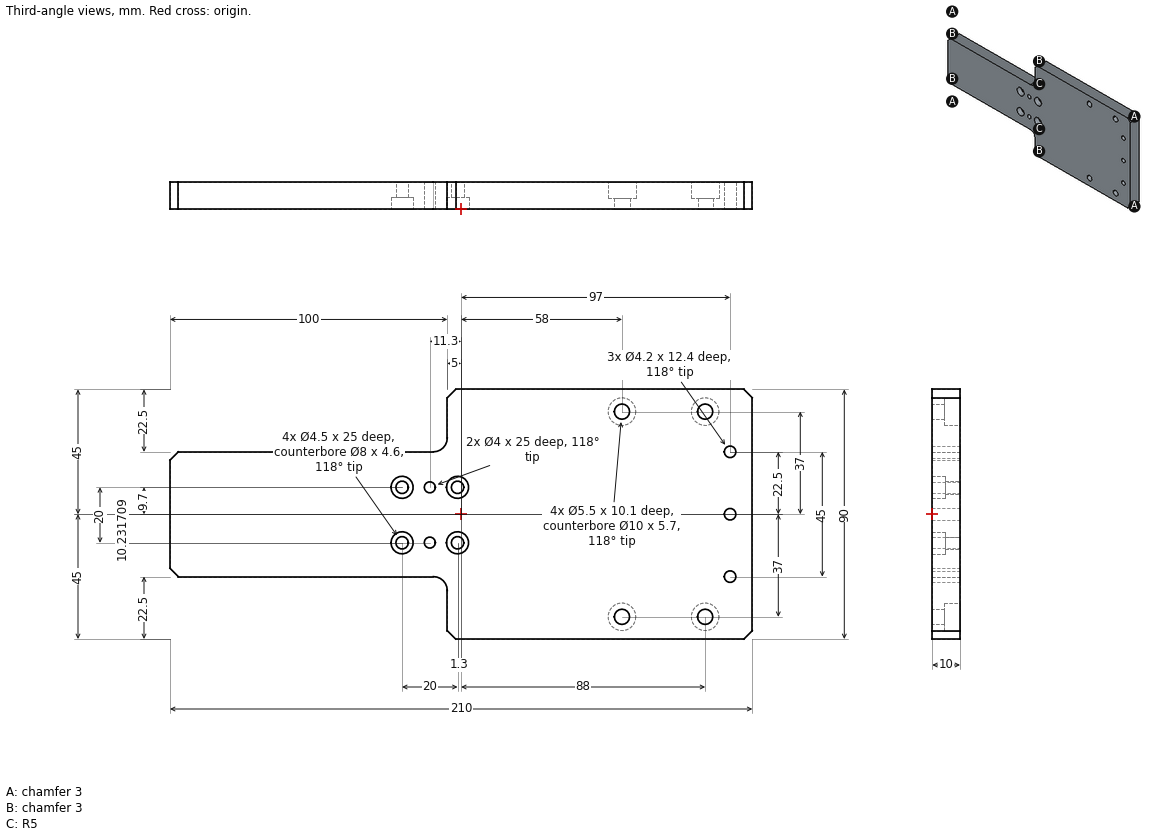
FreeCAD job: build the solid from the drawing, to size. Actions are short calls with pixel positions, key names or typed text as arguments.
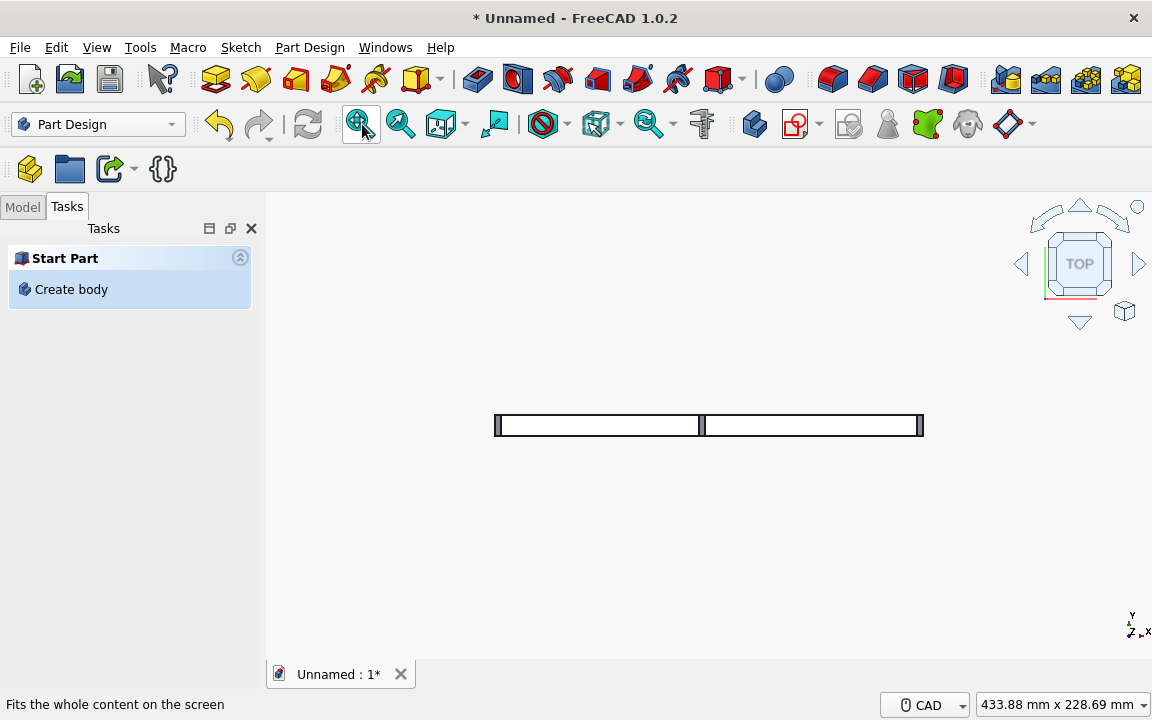
scroll(699, 424, up, 4)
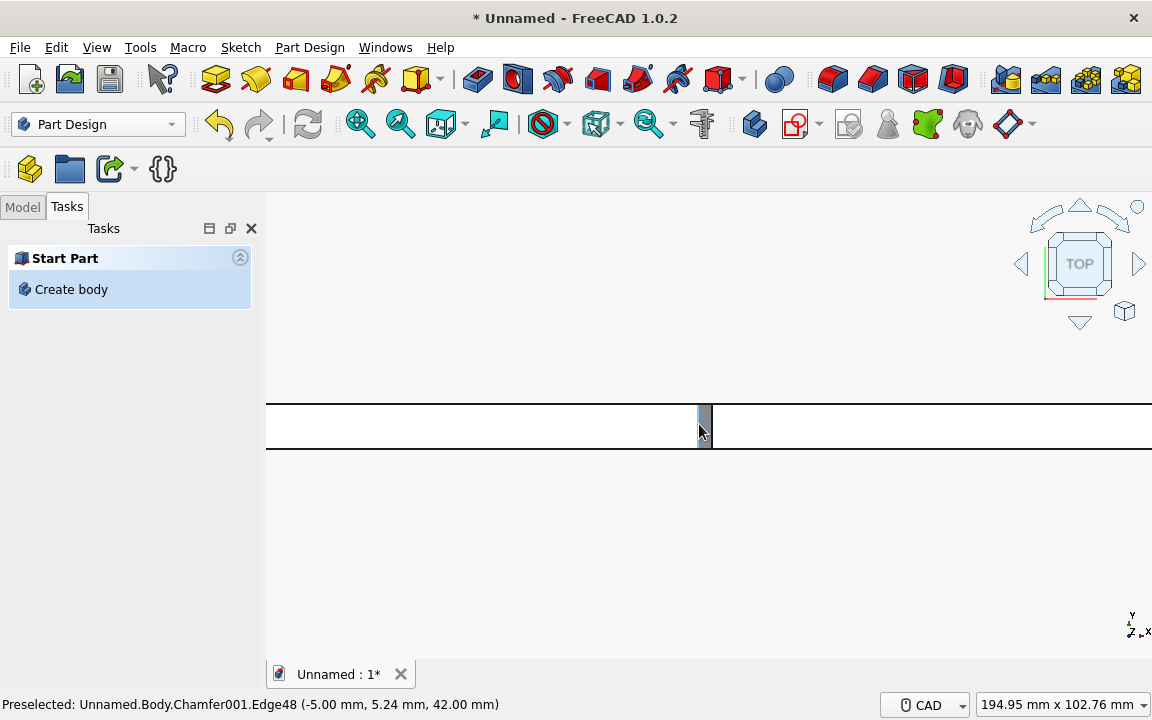
click(362, 124)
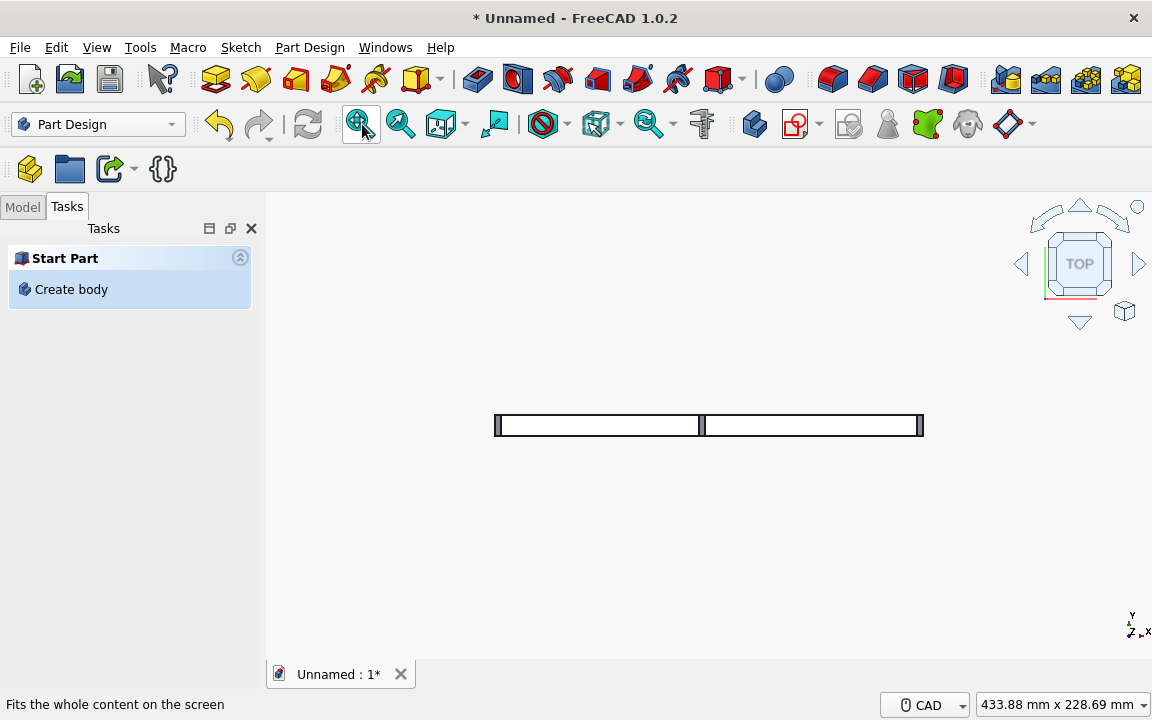
key(1)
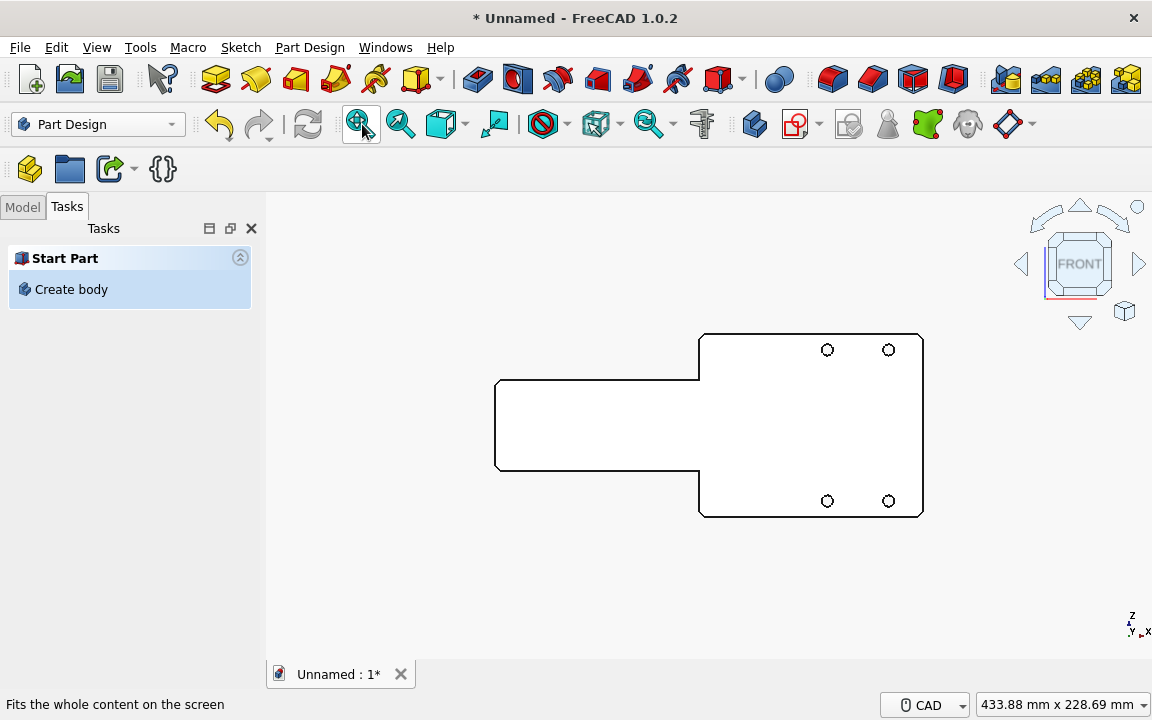
scroll(699, 379, up, 4)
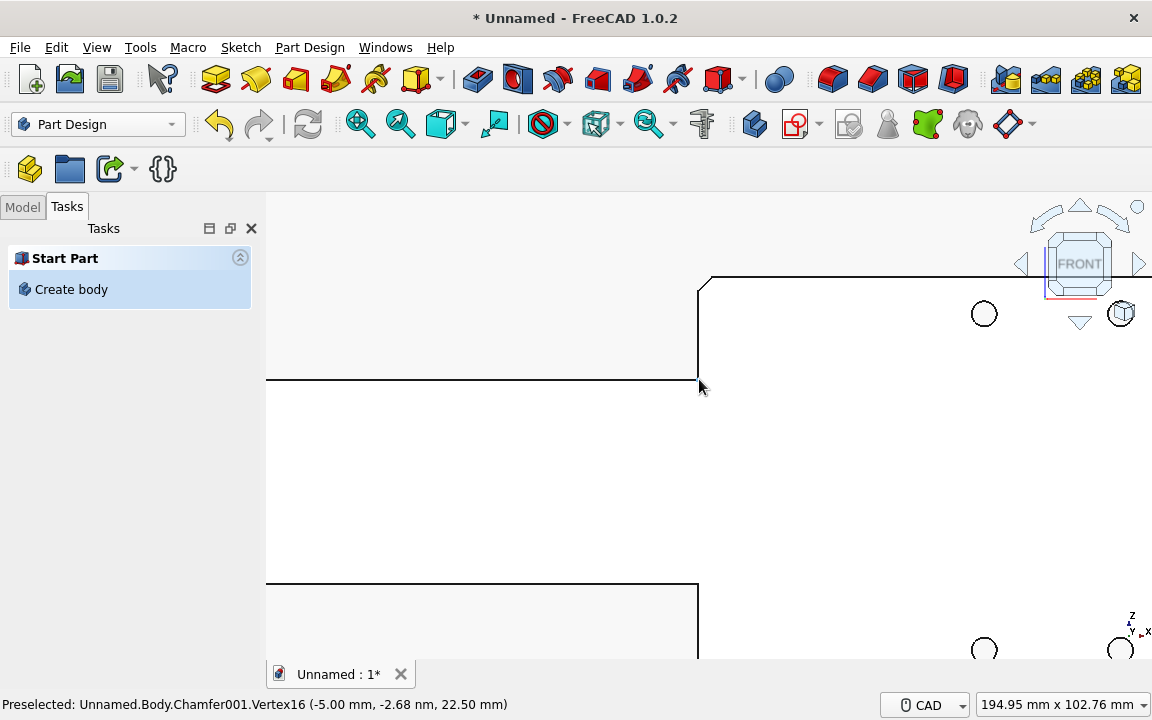
click(362, 124)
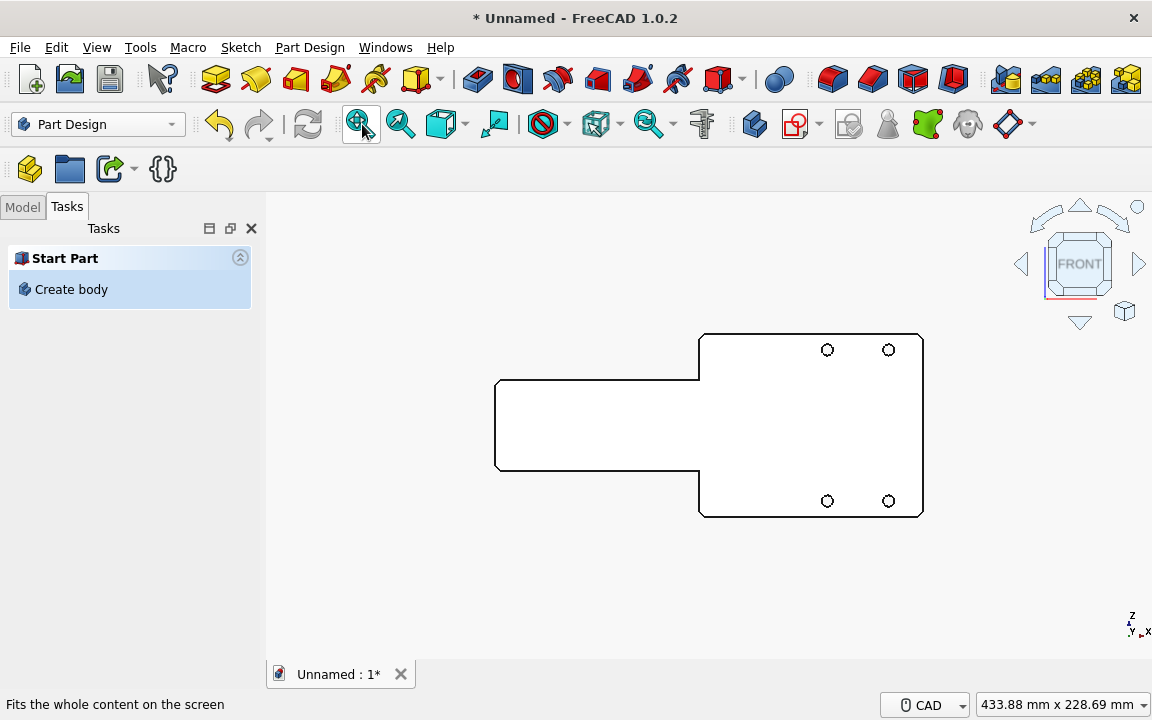
key(3)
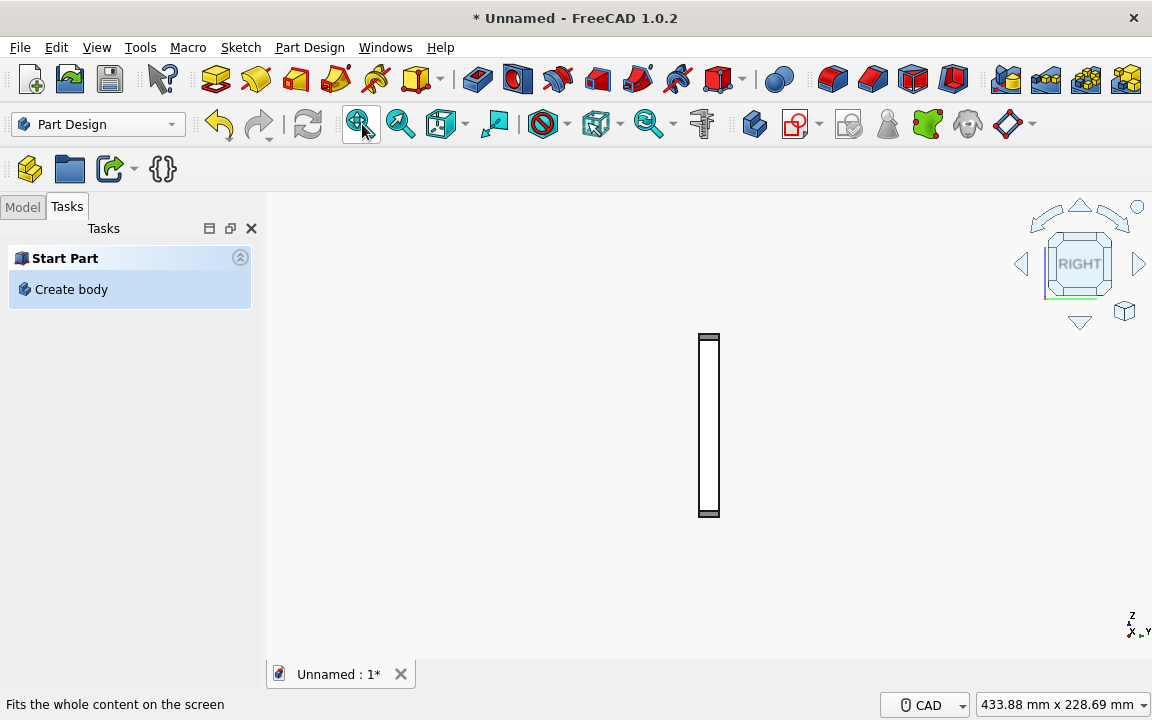
click(362, 124)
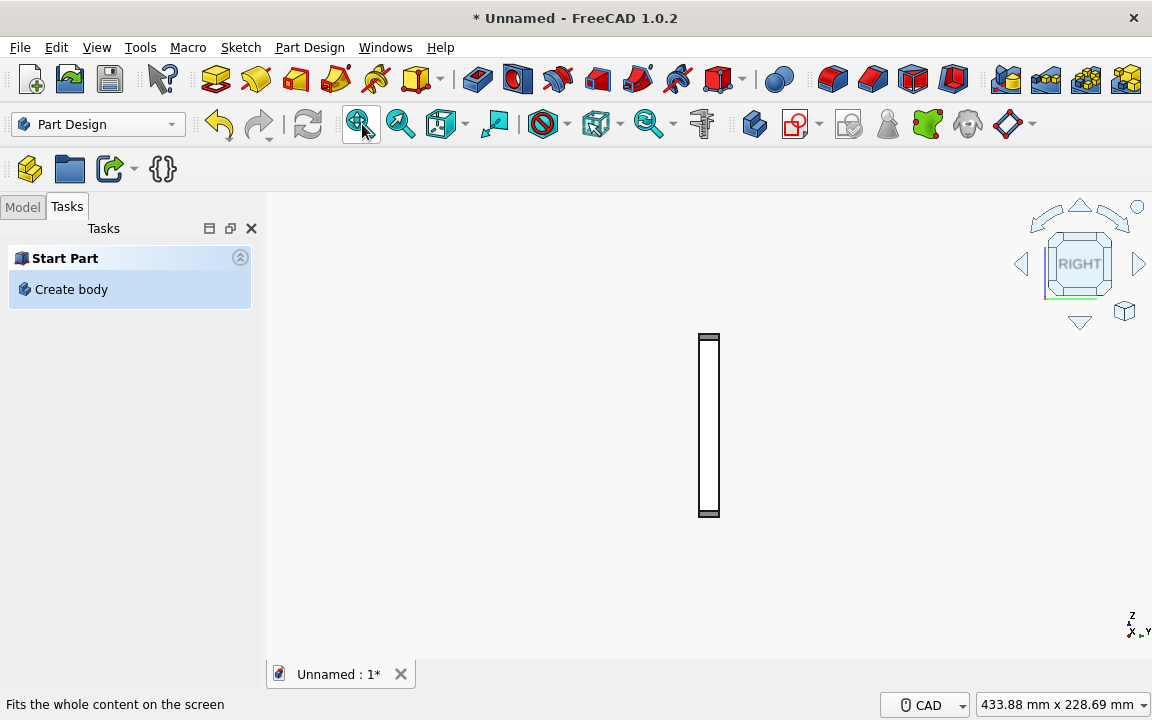
scroll(709, 379, up, 4)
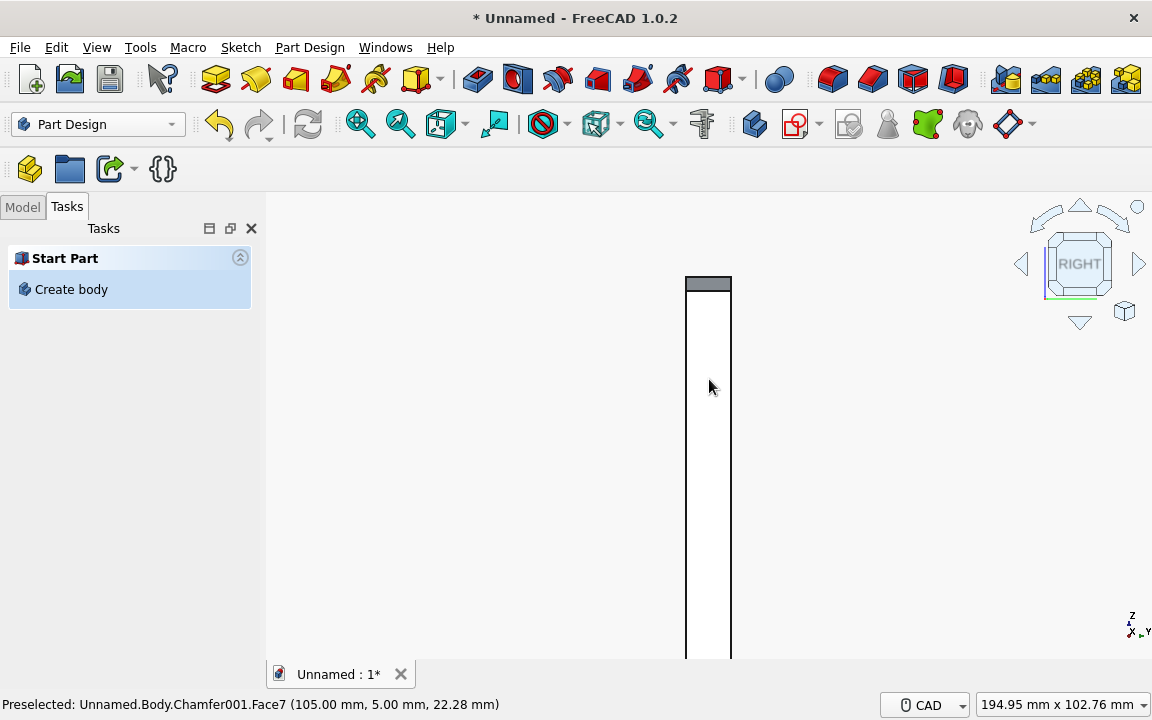
click(362, 124)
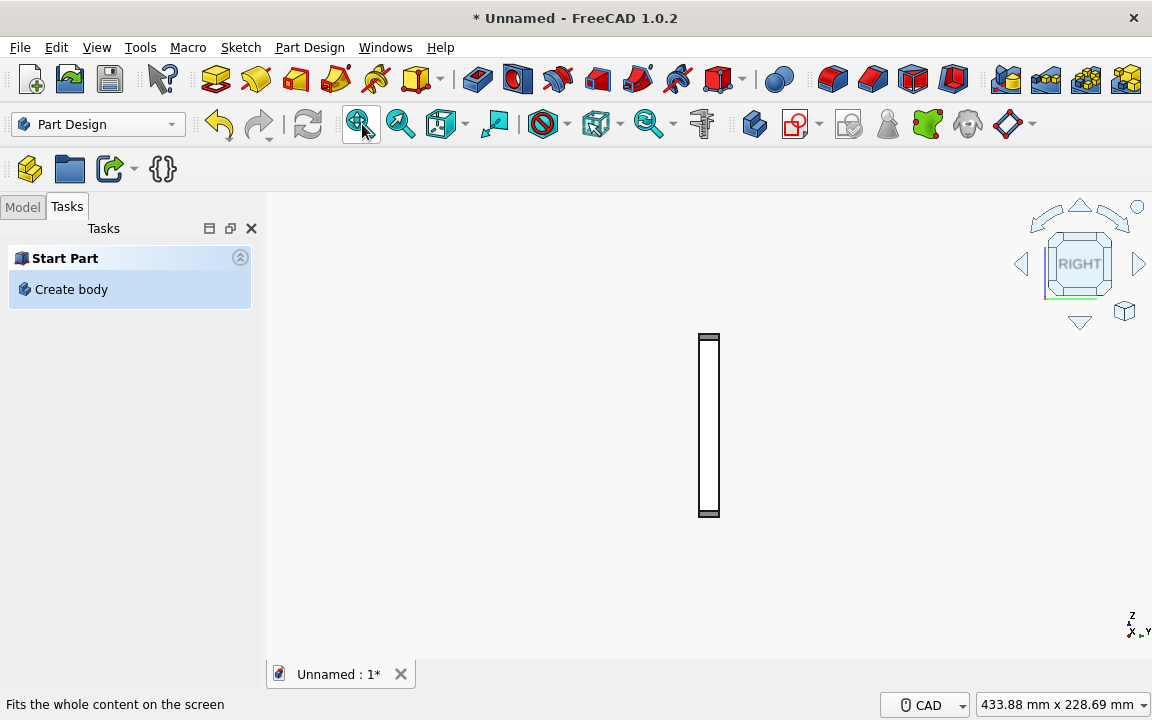
key(5)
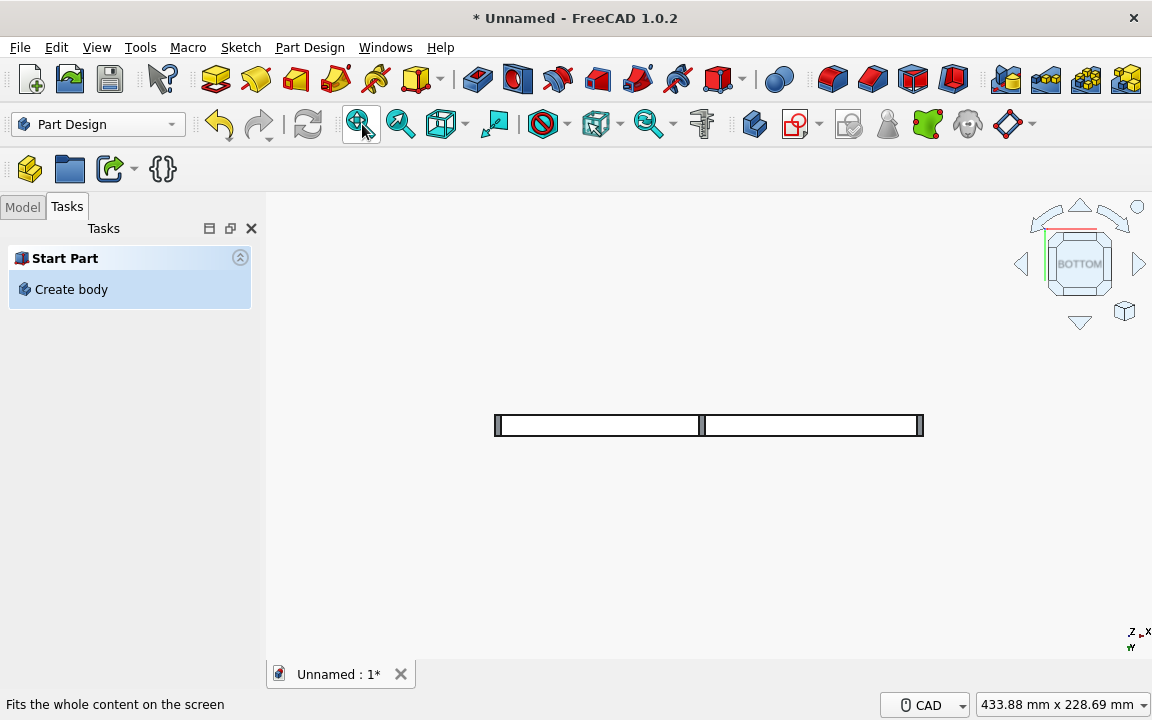
scroll(699, 424, up, 4)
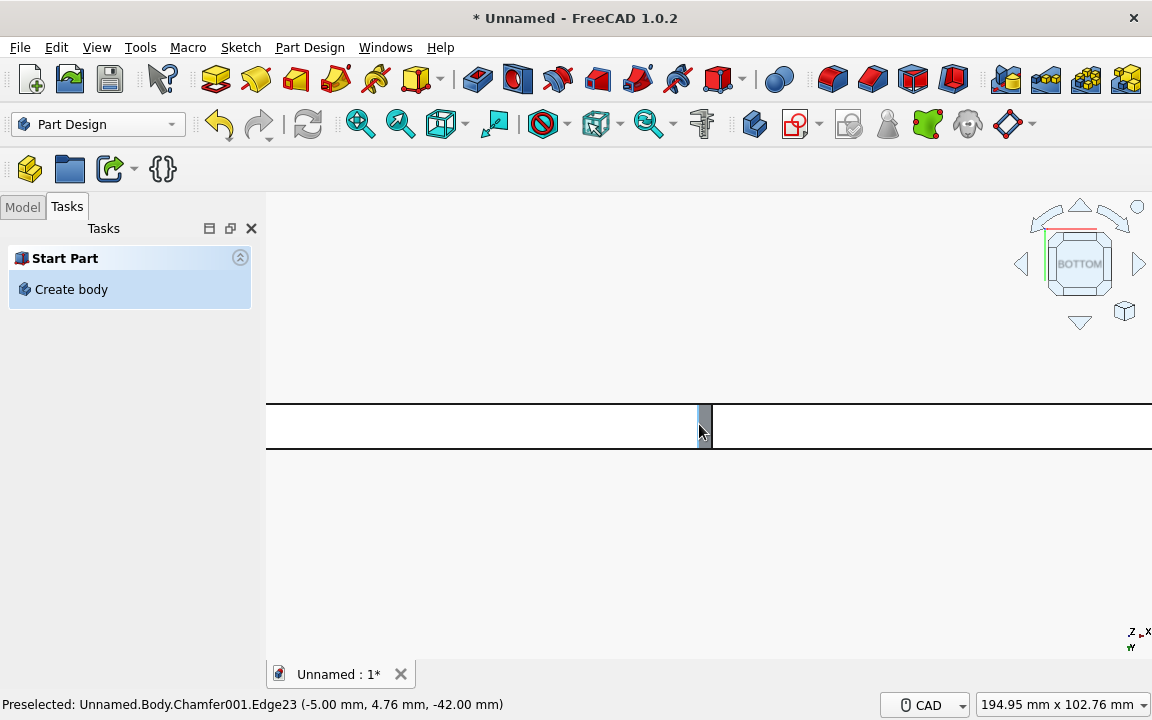
click(362, 124)